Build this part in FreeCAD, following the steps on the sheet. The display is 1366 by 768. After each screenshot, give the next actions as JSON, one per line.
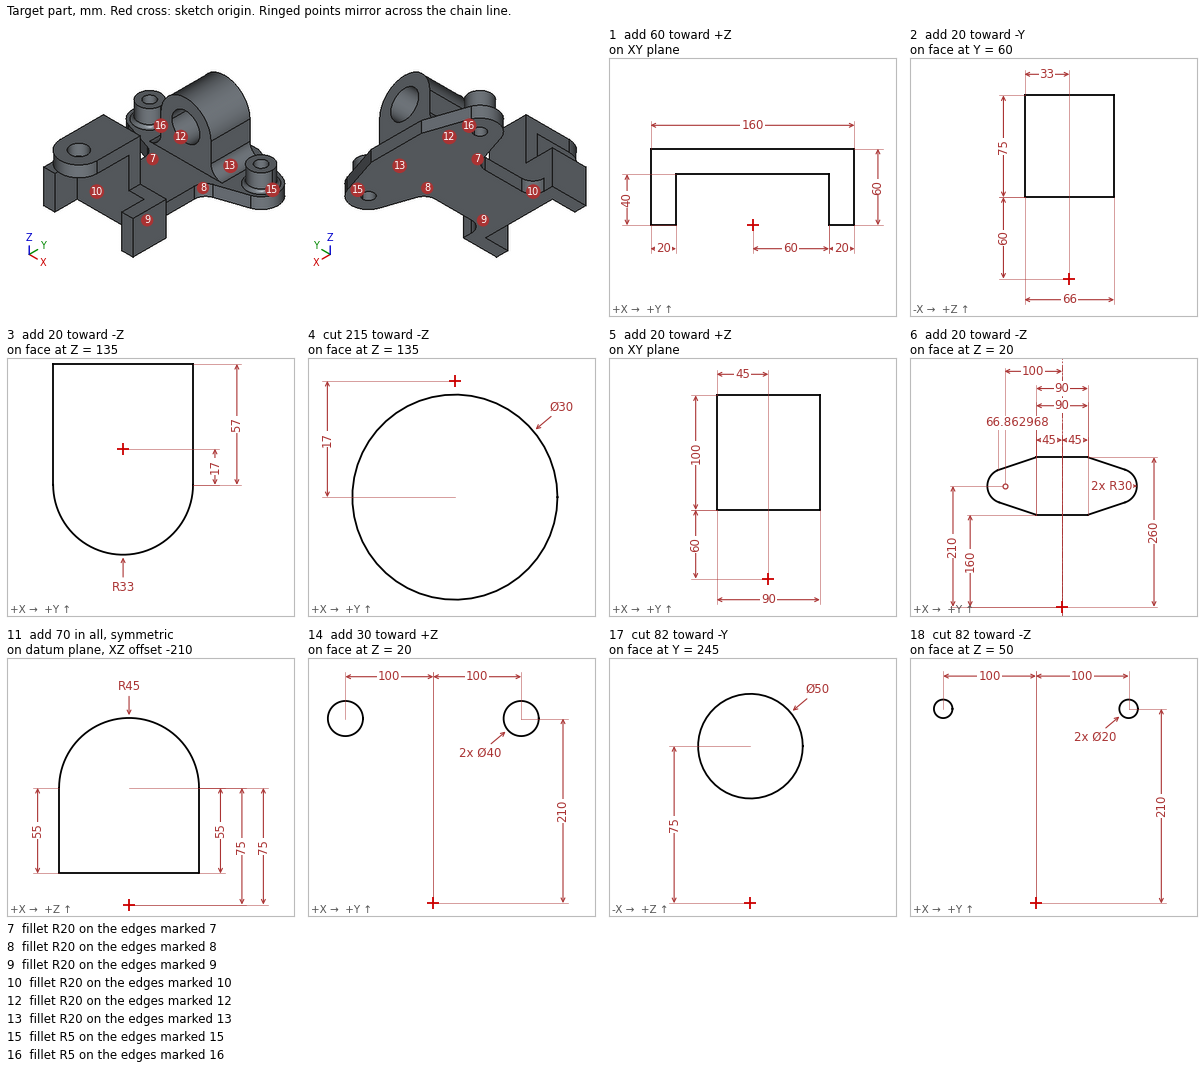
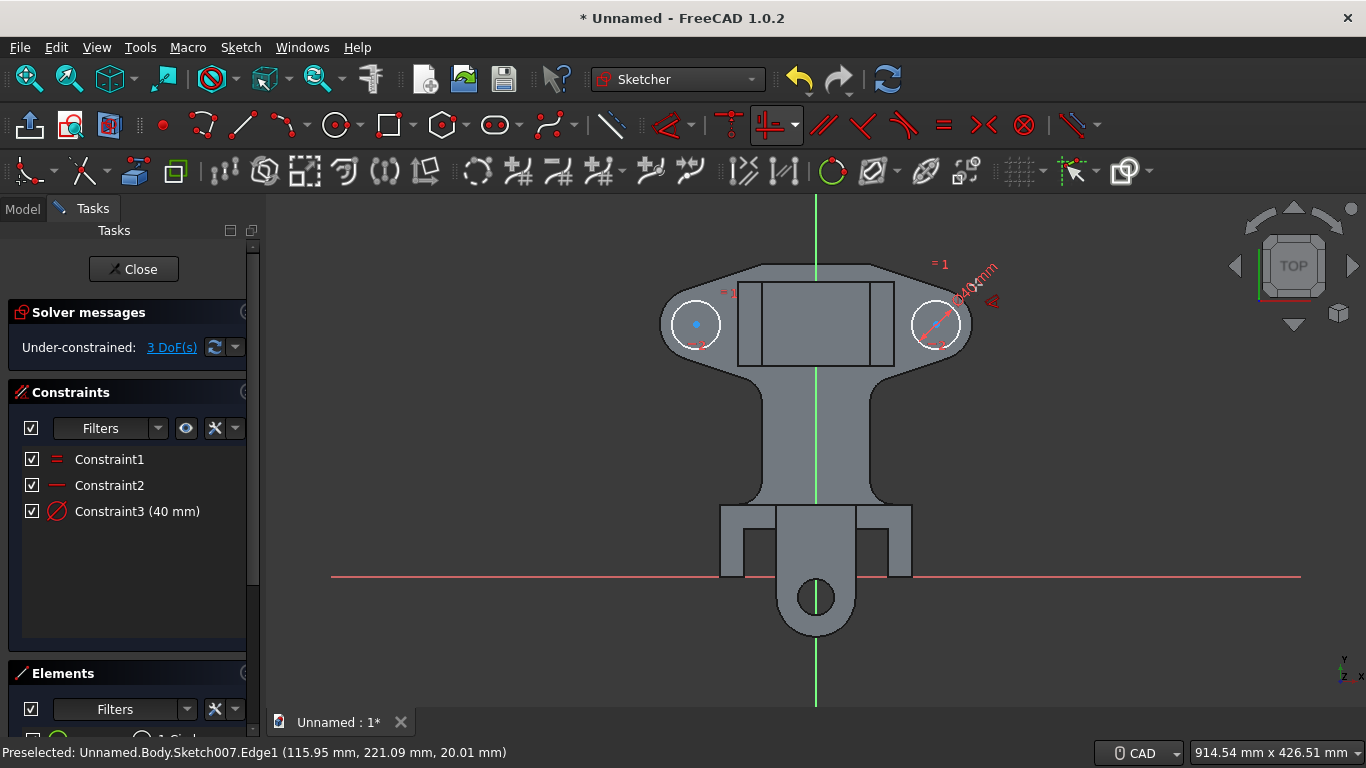
{"action": "left_click", "coordinate": [936, 325]}
{"action": "left_click", "coordinate": [876, 611]}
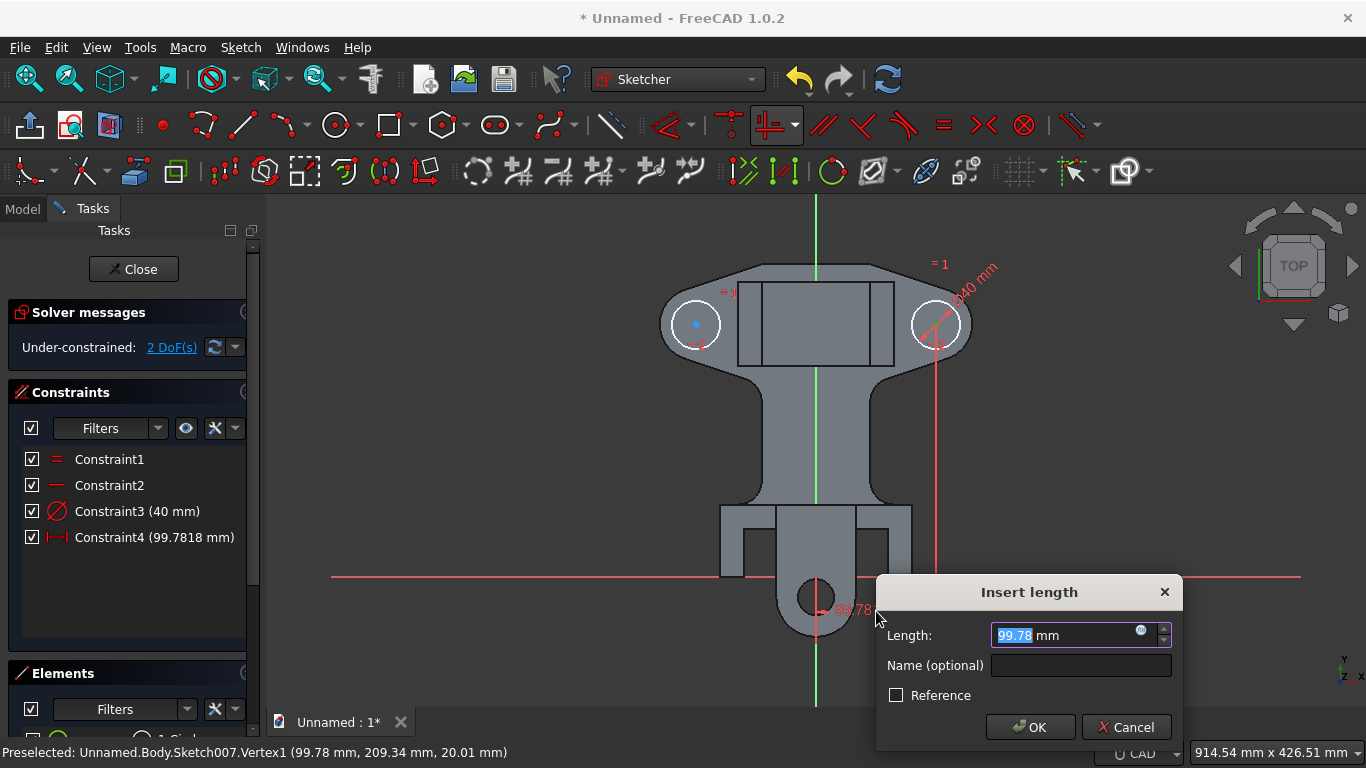
{"action": "type", "text": "100"}
{"action": "key", "text": "Return"}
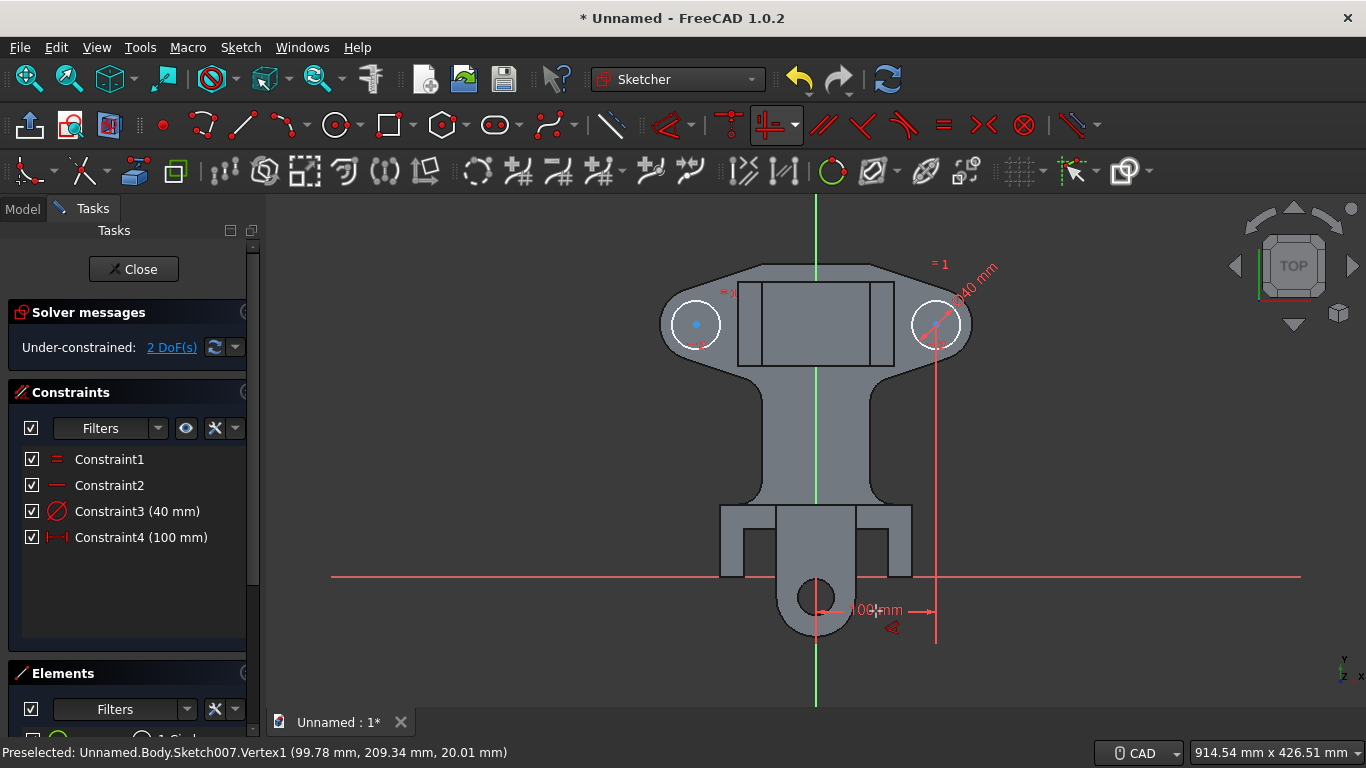
{"action": "left_click", "coordinate": [936, 325]}
{"action": "left_click", "coordinate": [970, 451]}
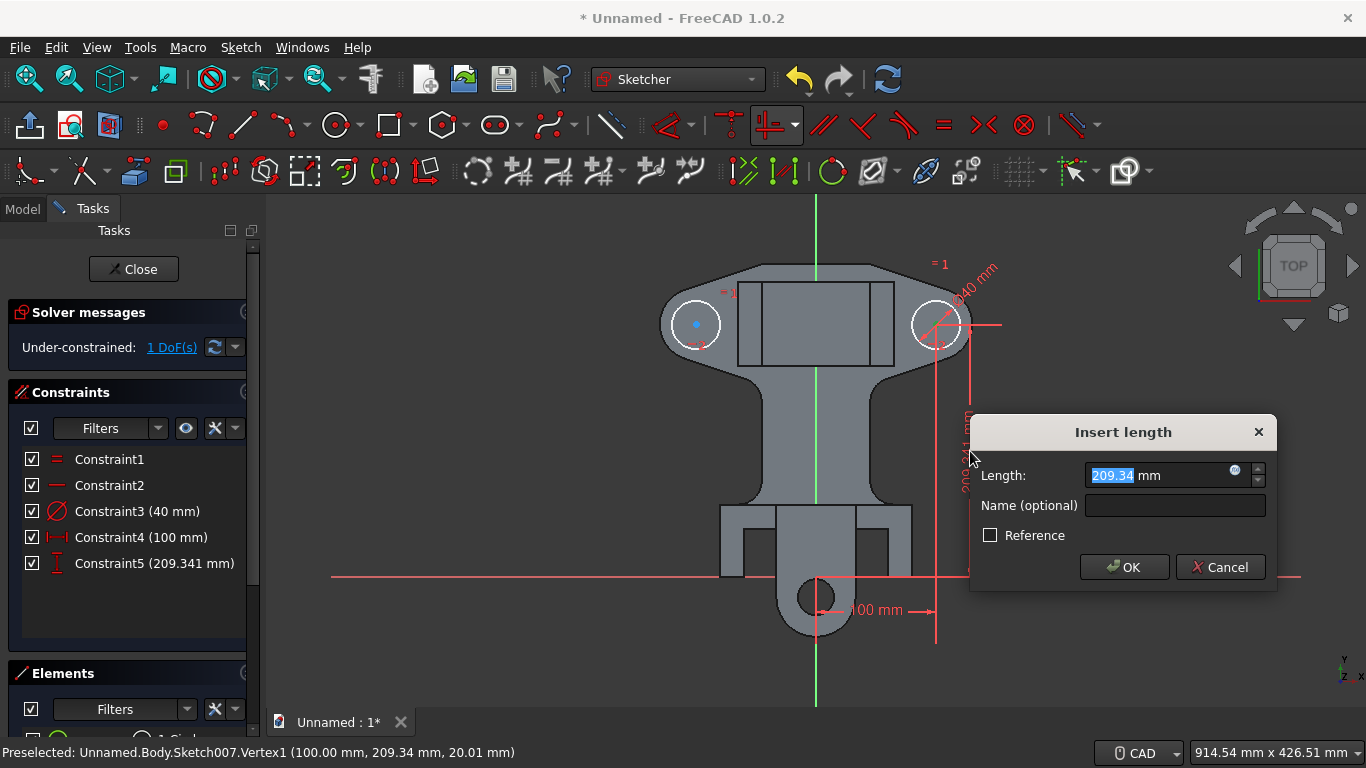
{"action": "type", "text": "210"}
{"action": "key", "text": "Return"}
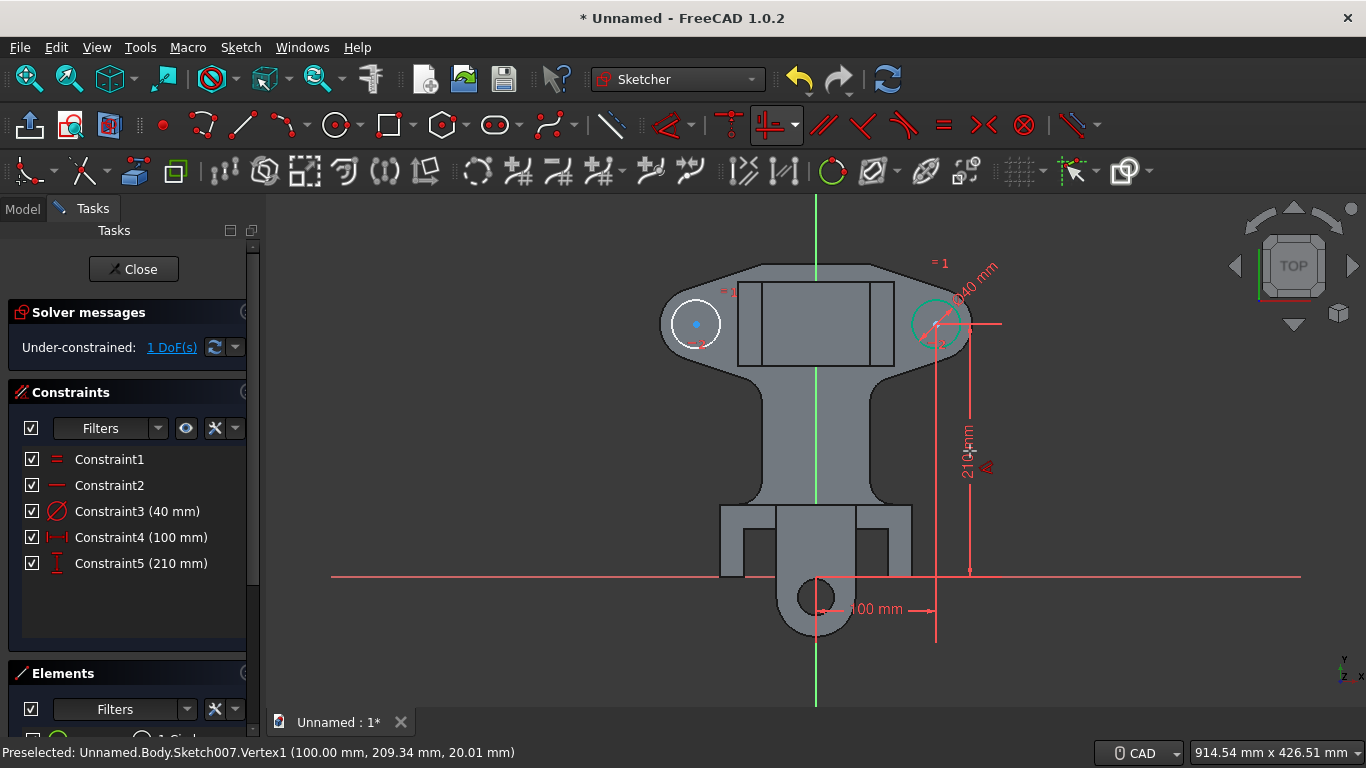
{"action": "left_click", "coordinate": [696, 324]}
{"action": "left_click", "coordinate": [756, 611]}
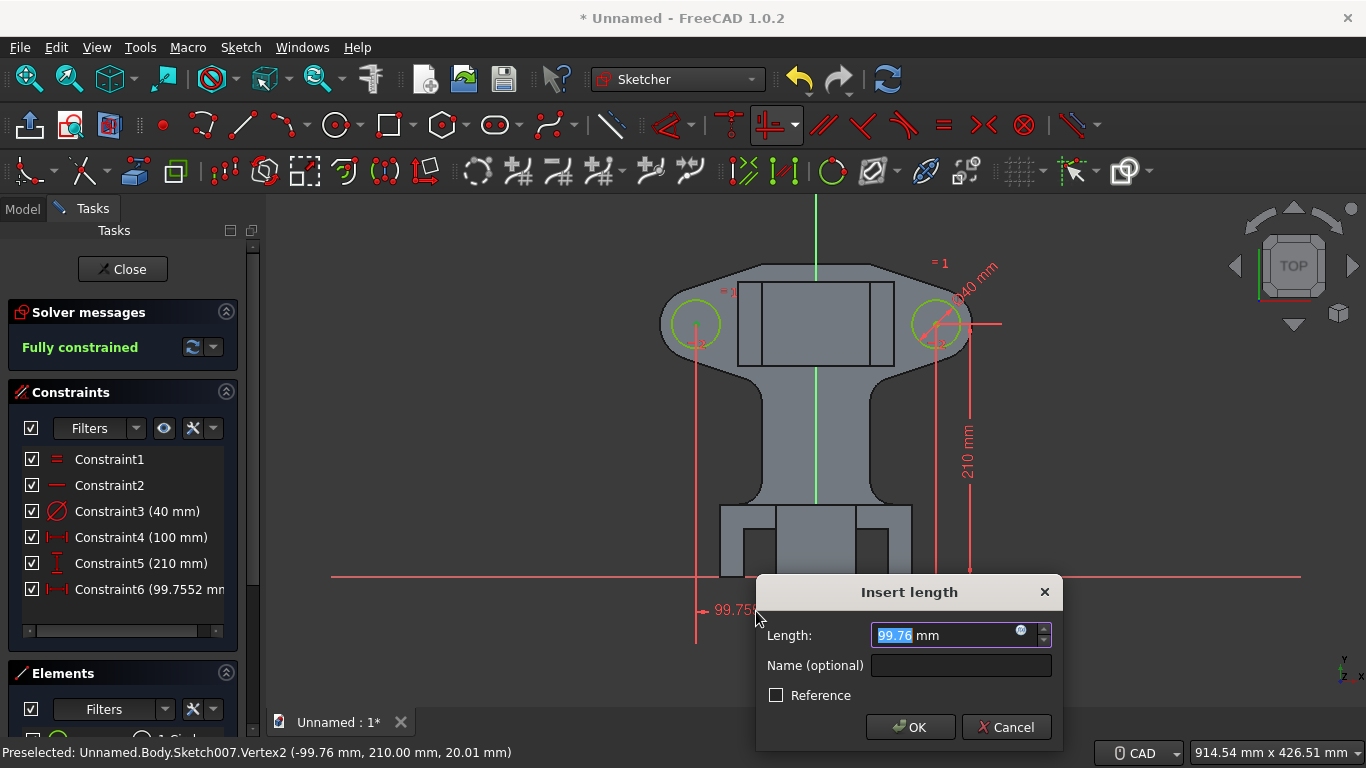
{"action": "type", "text": "100"}
{"action": "key", "text": "Return"}
{"action": "key", "text": "Escape"}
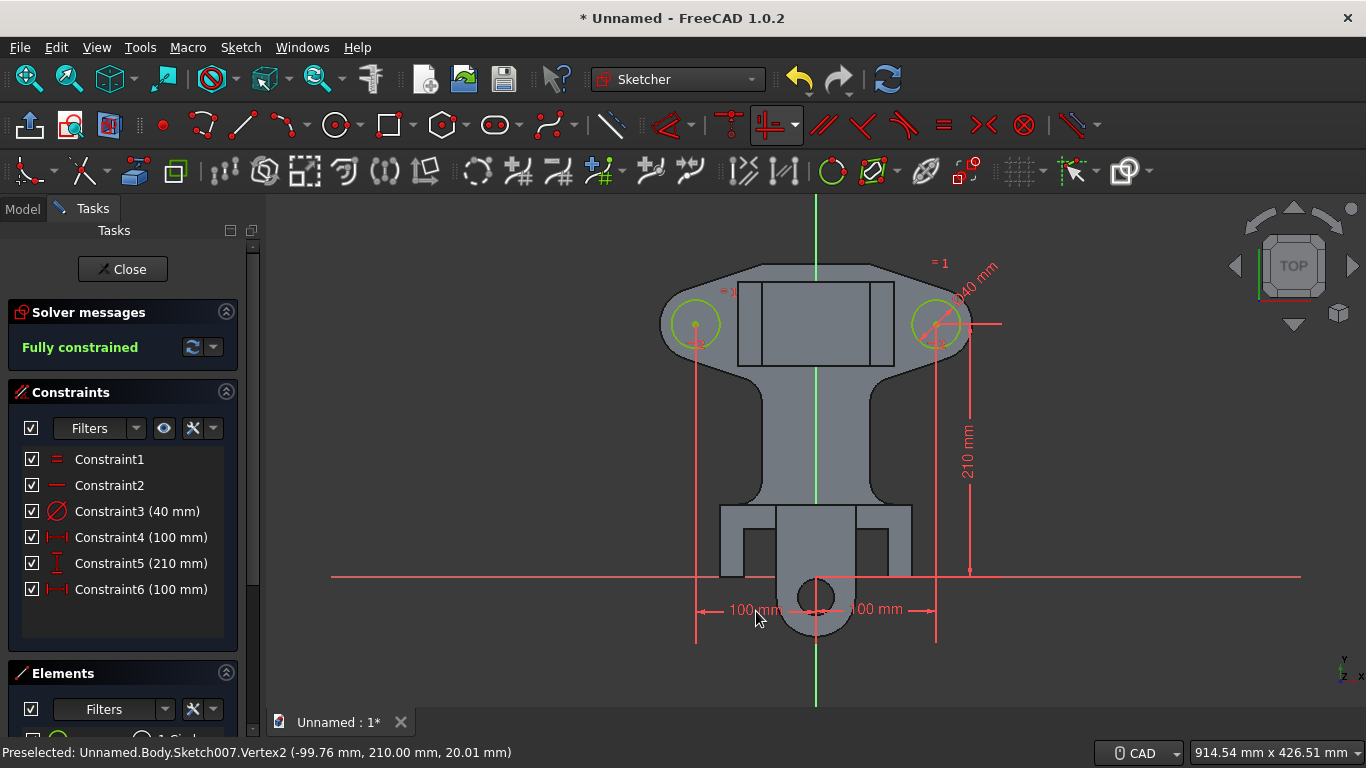
{"action": "left_click", "coordinate": [123, 269]}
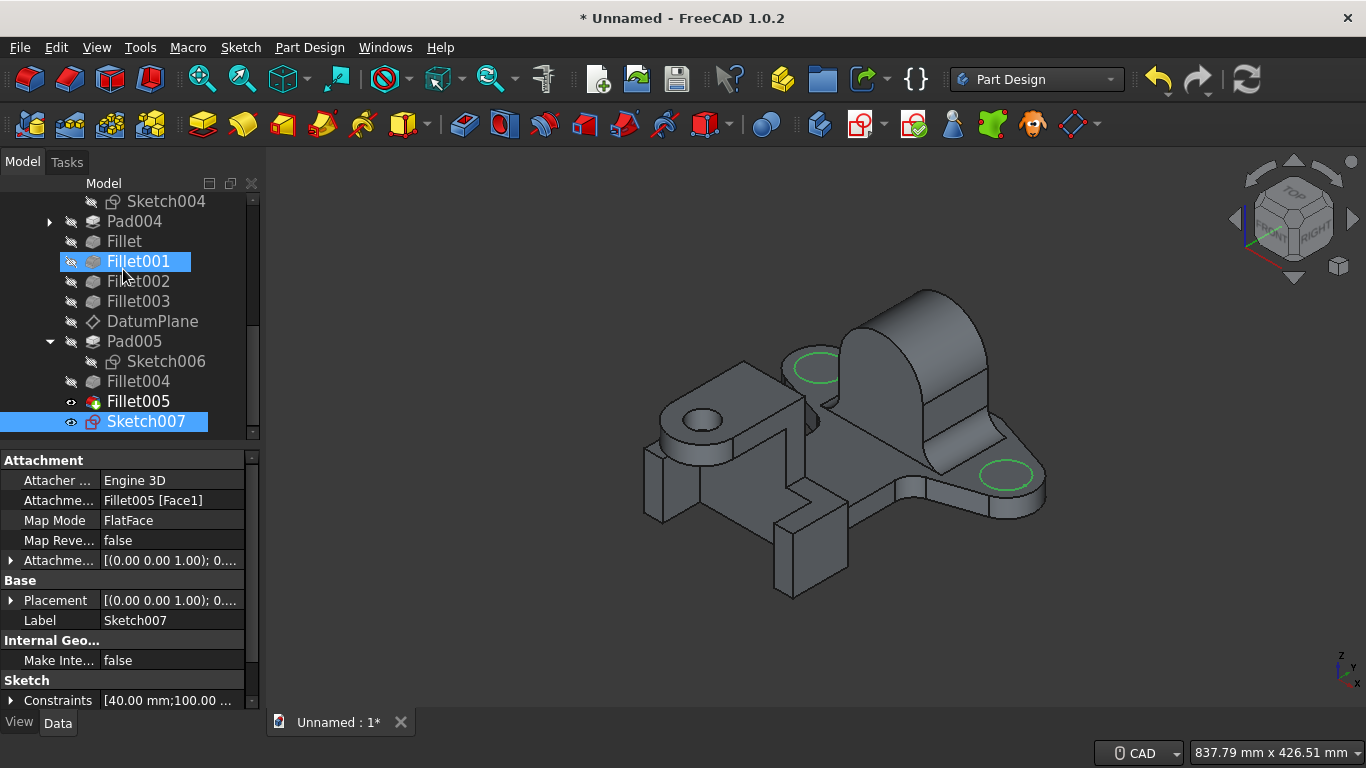
{"action": "left_click", "coordinate": [204, 124]}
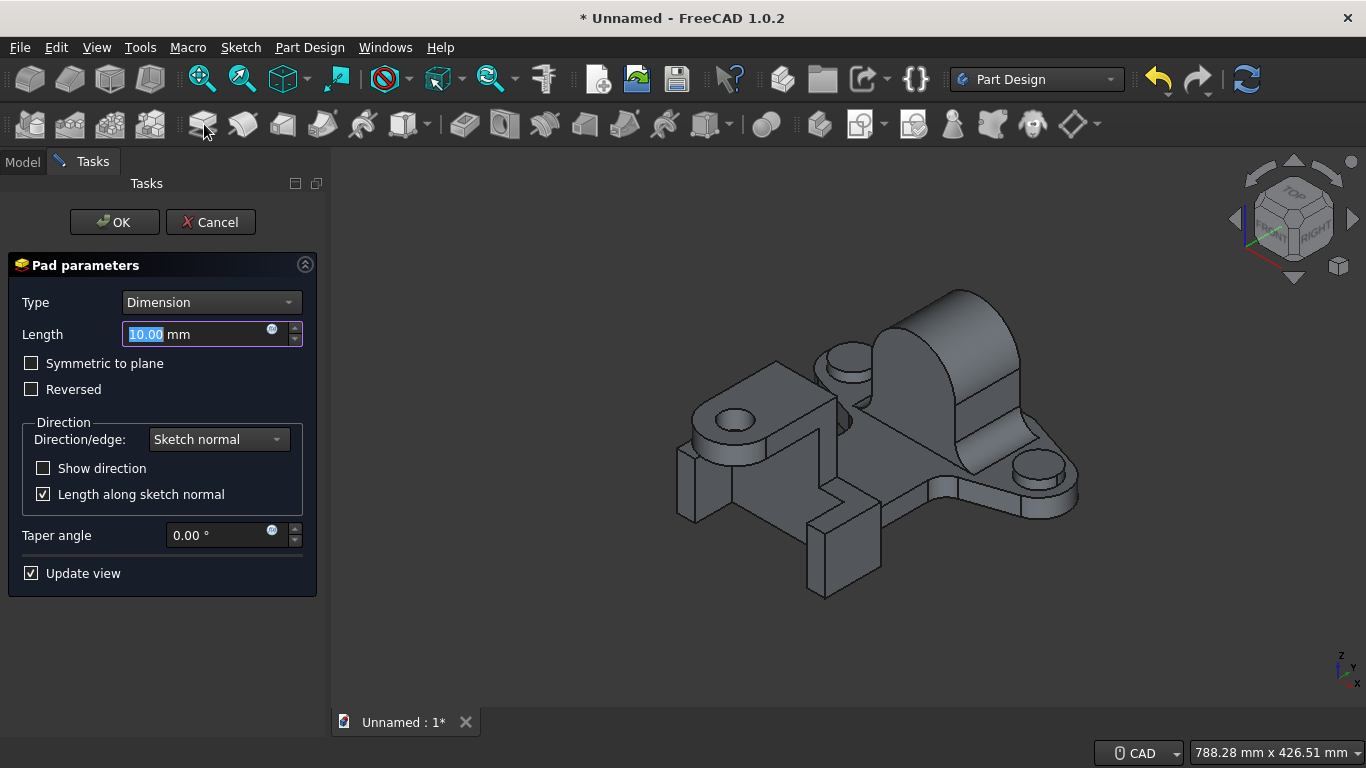
{"action": "type", "text": "30"}
{"action": "key", "text": "Tab"}